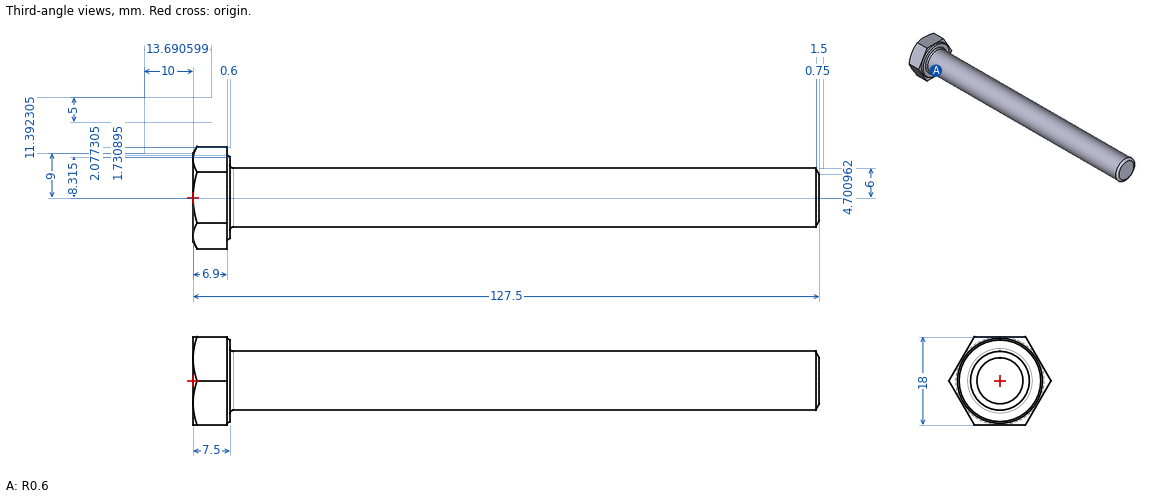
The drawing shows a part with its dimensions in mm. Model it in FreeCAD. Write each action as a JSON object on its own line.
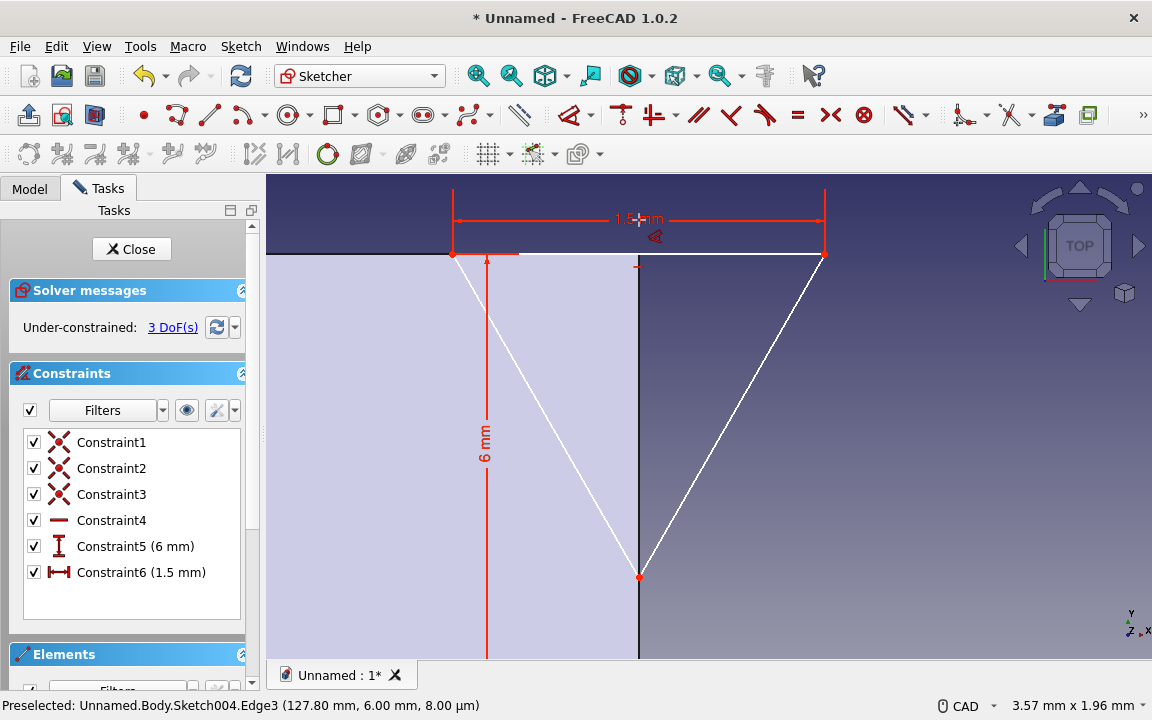
{"action": "left_click", "coordinate": [509, 351]}
{"action": "left_click", "coordinate": [546, 612]}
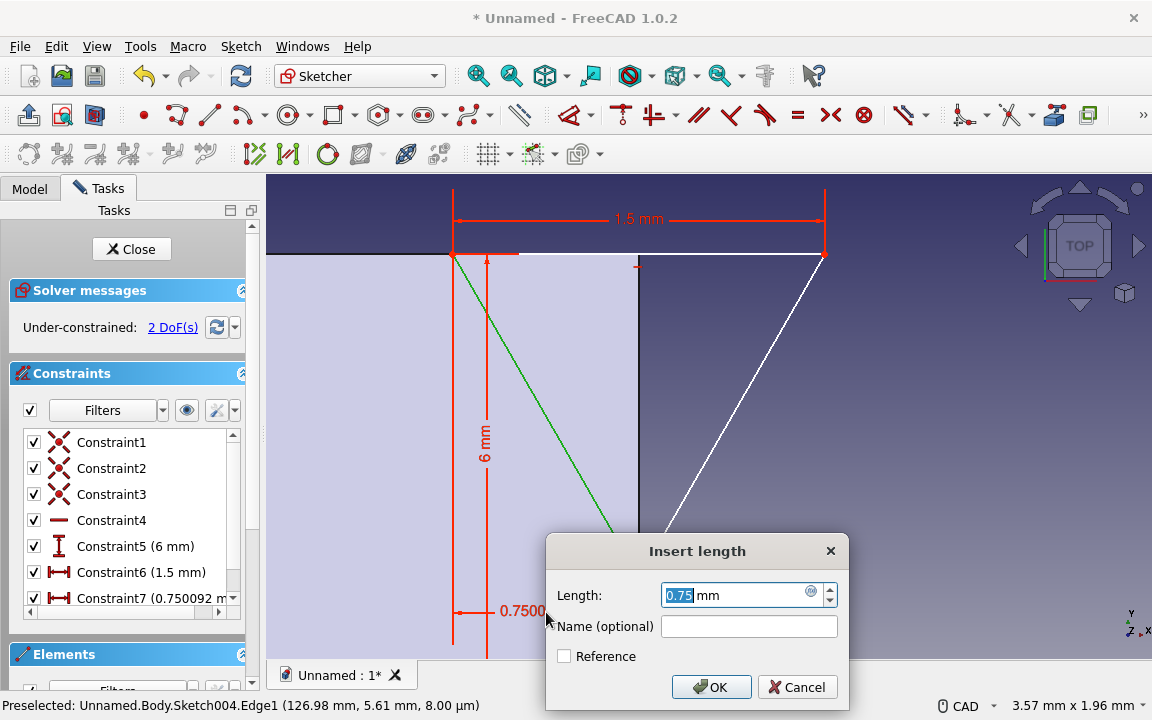
{"action": "type", "text": "0.75"}
{"action": "key", "text": "Return"}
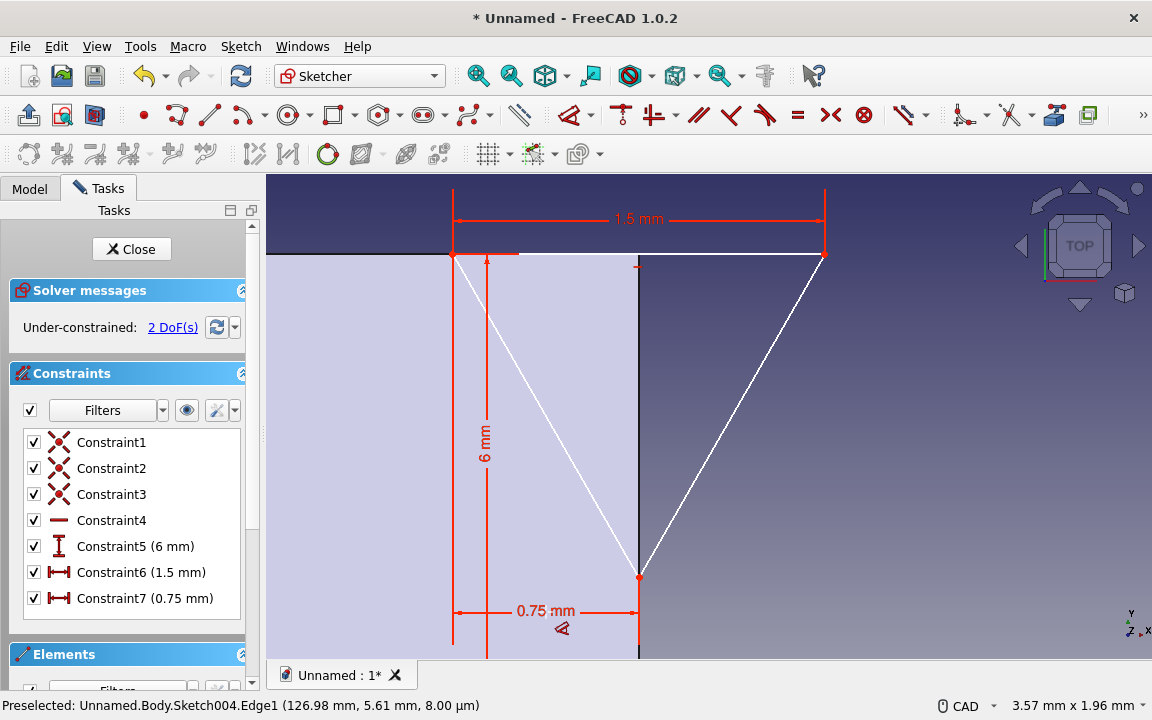
{"action": "left_click", "coordinate": [639, 578]}
{"action": "left_click", "coordinate": [466, 544]}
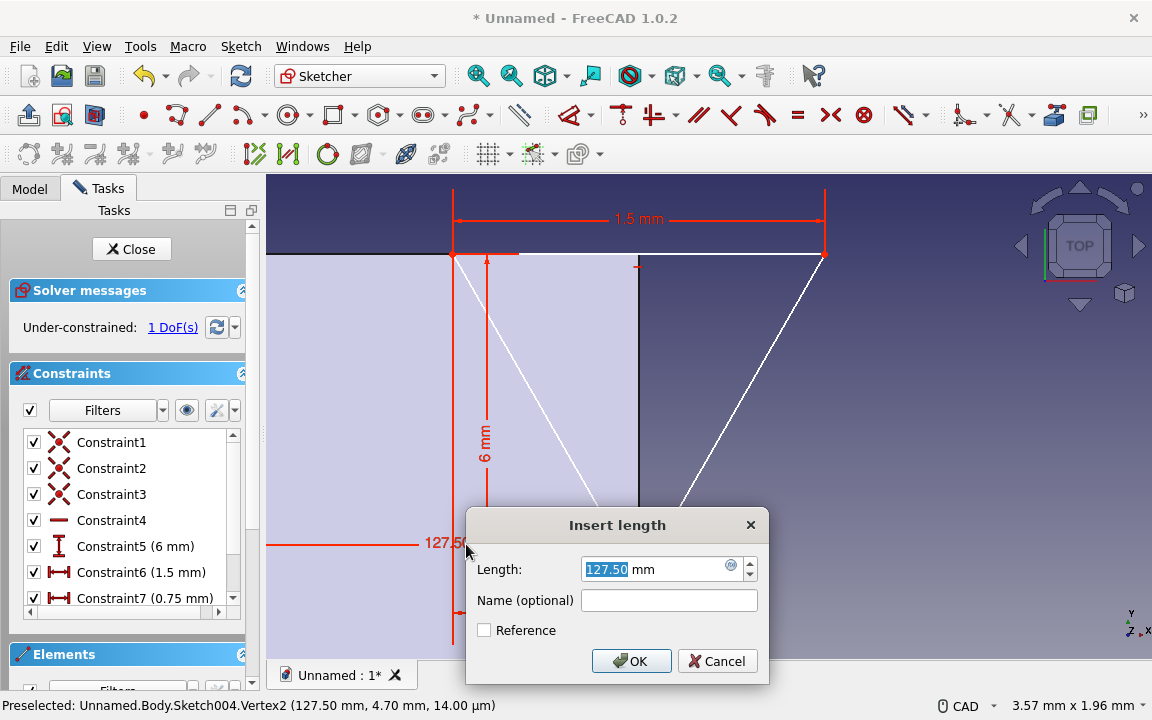
{"action": "type", "text": "127.5"}
{"action": "key", "text": "Return"}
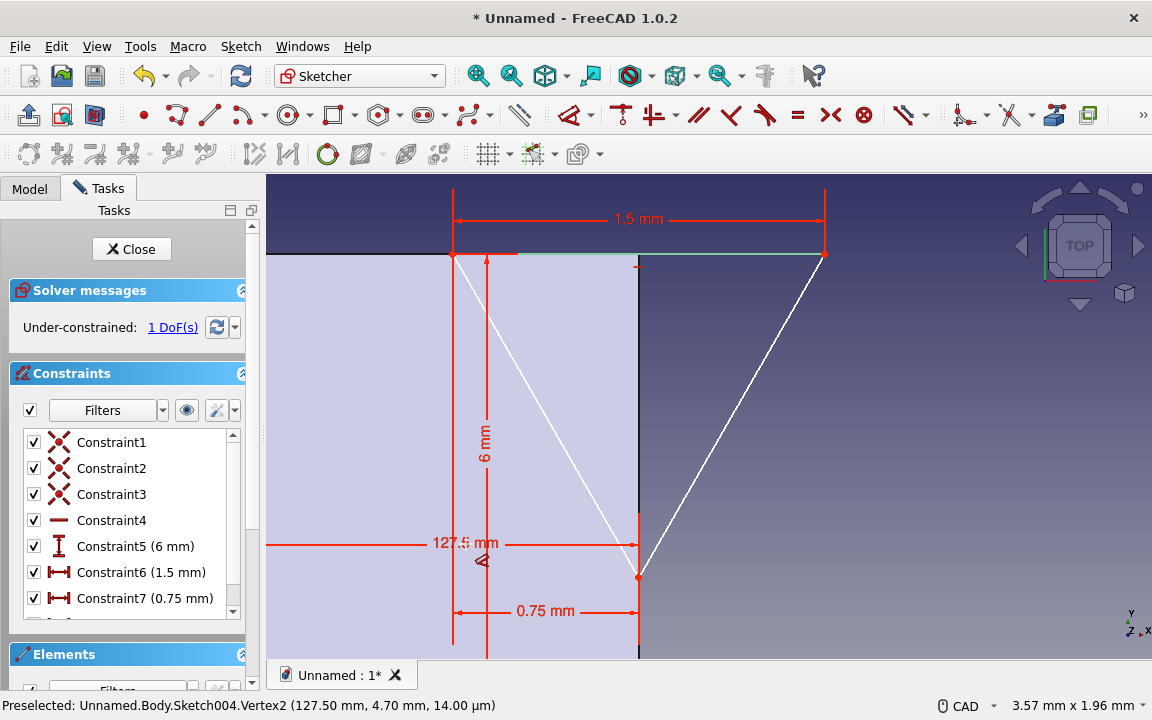
{"action": "left_click", "coordinate": [639, 578]}
{"action": "left_click", "coordinate": [673, 604]}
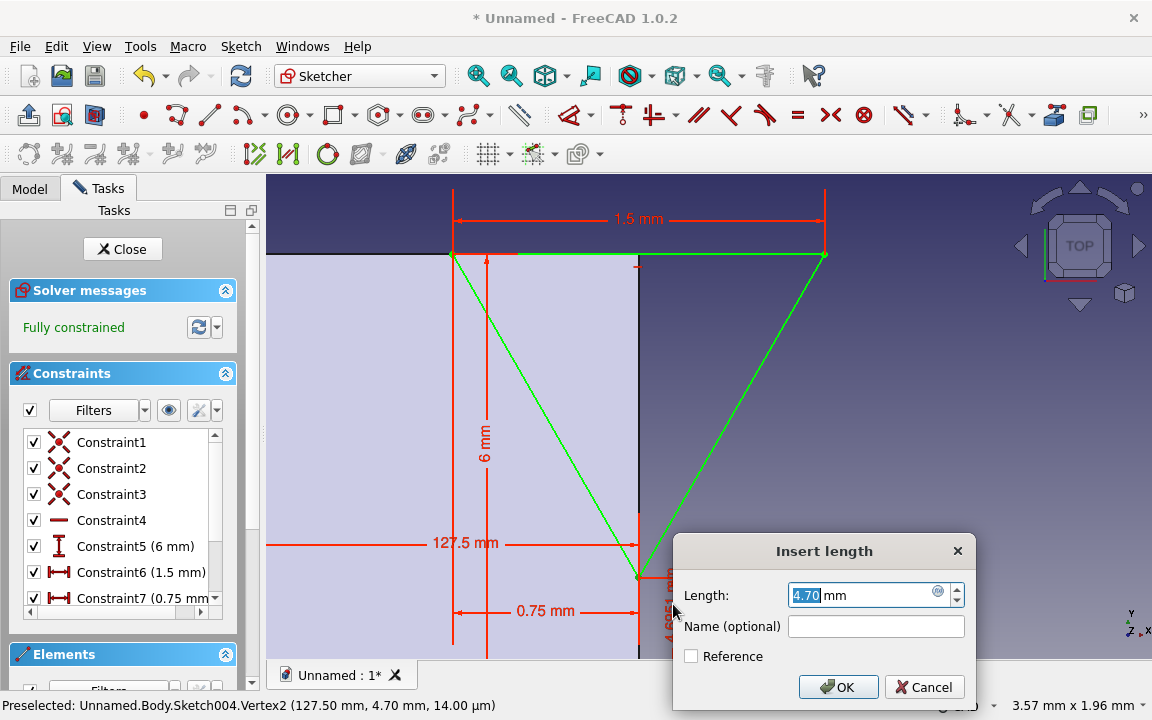
{"action": "type", "text": "4.700962"}
{"action": "key", "text": "Return"}
{"action": "key", "text": "Escape"}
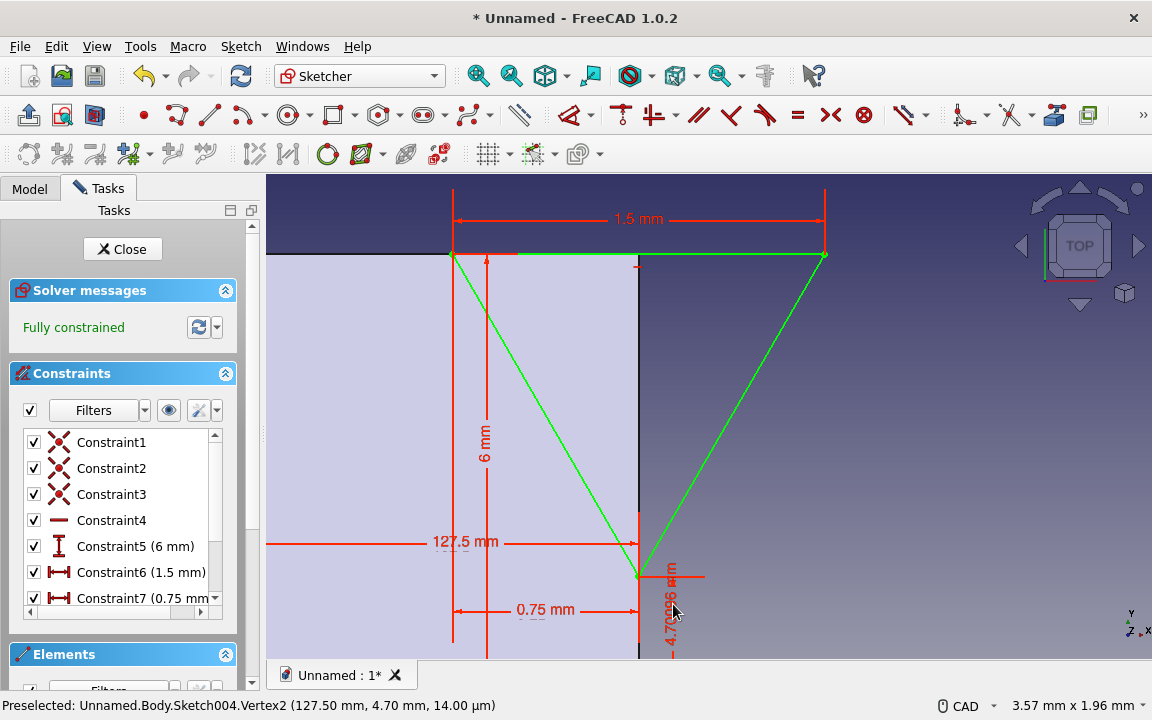
{"action": "left_click", "coordinate": [123, 249]}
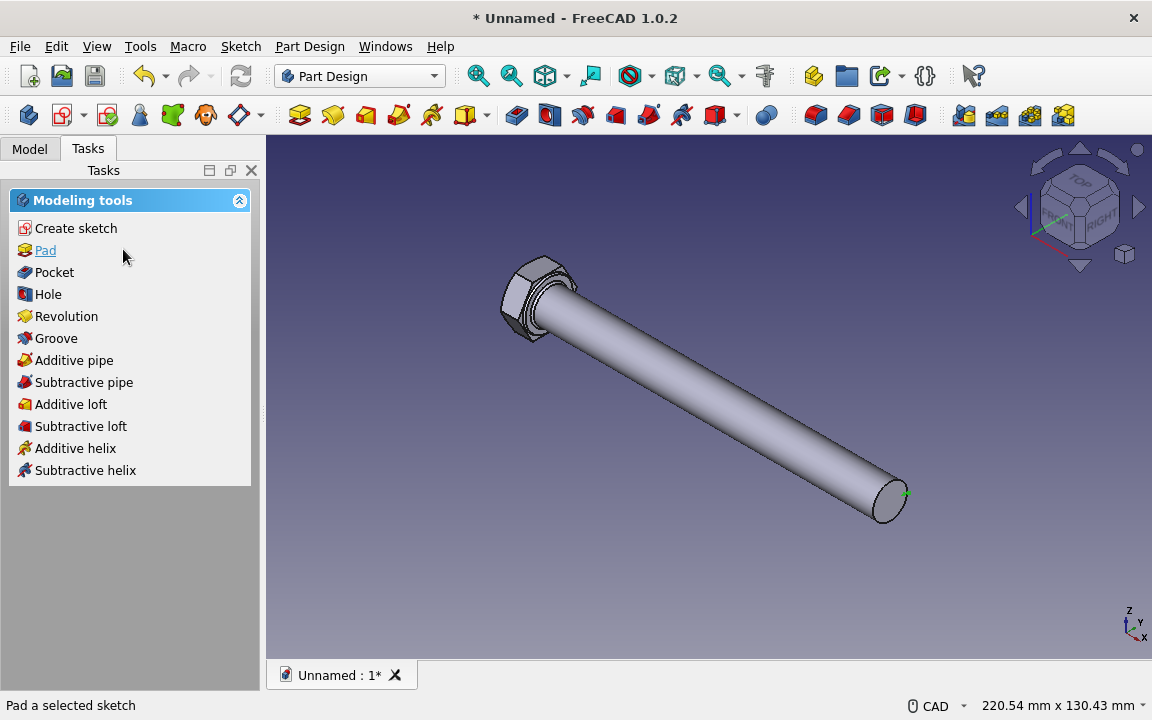
{"action": "left_click", "coordinate": [583, 116]}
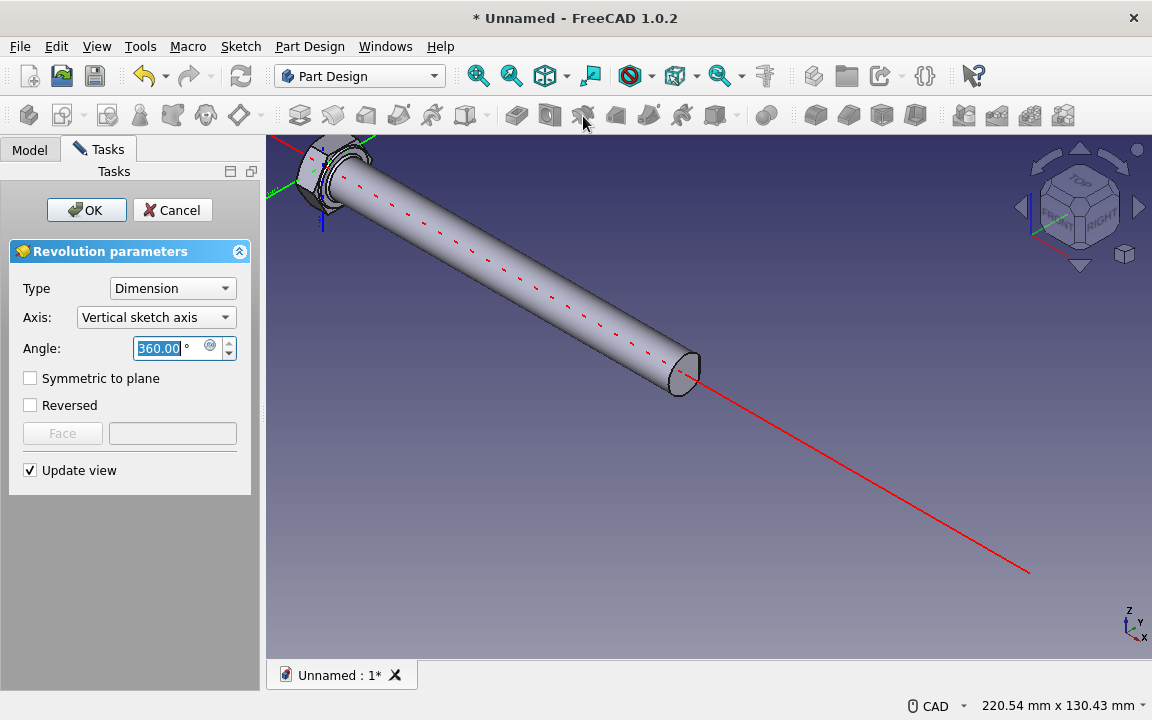
{"action": "left_click", "coordinate": [157, 318]}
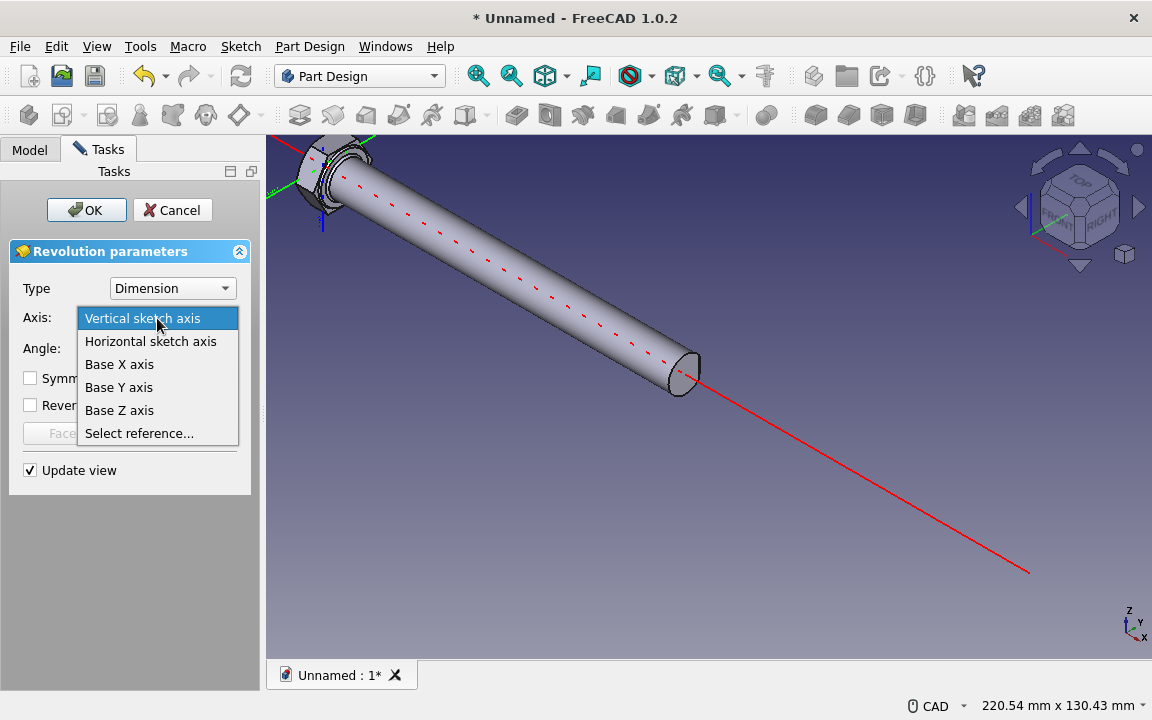
{"action": "left_click", "coordinate": [156, 342]}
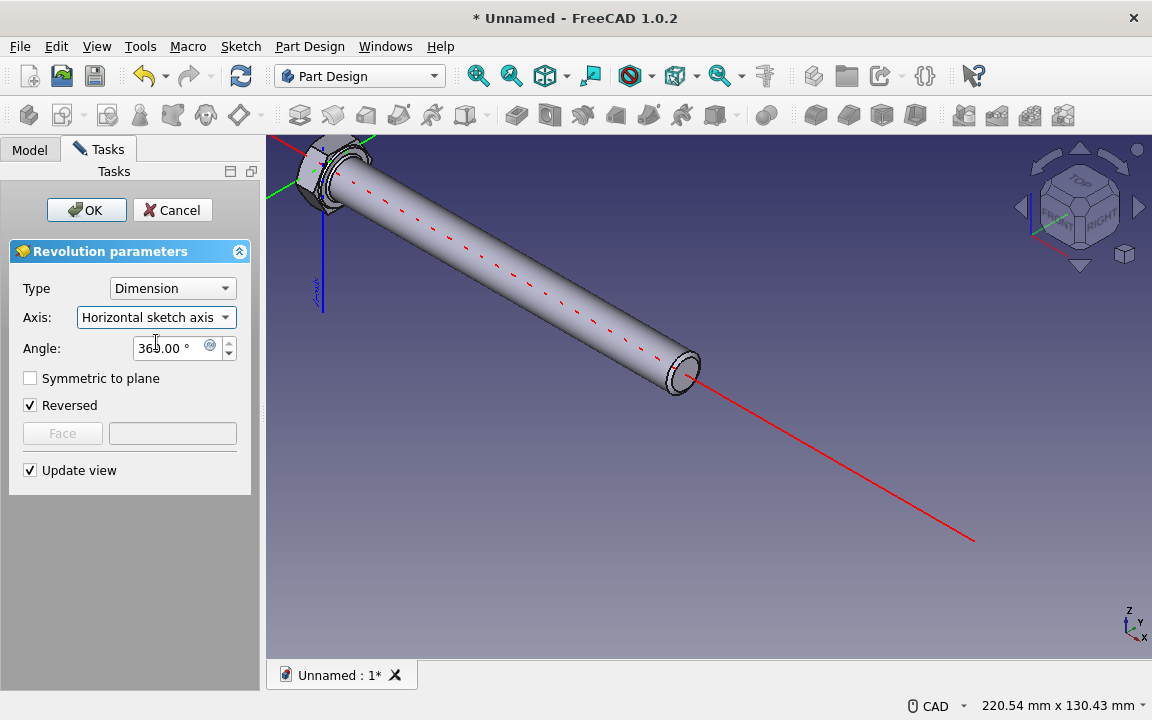
{"action": "left_click", "coordinate": [87, 210]}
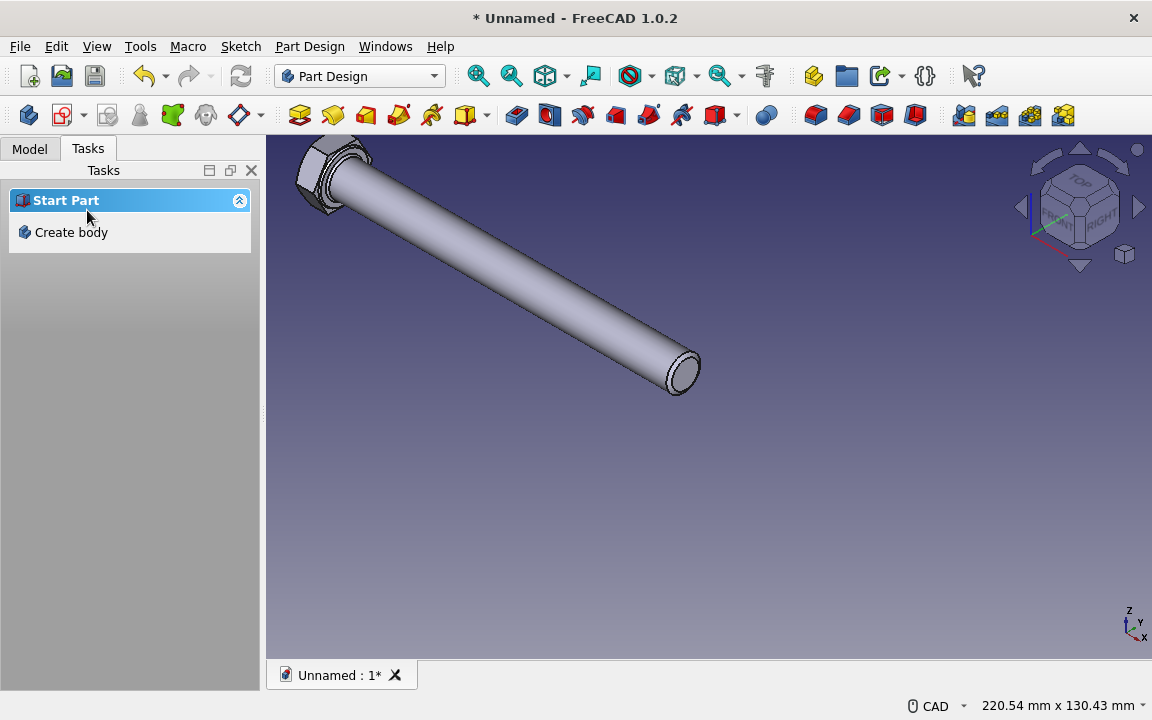
{"action": "left_click", "coordinate": [479, 76]}